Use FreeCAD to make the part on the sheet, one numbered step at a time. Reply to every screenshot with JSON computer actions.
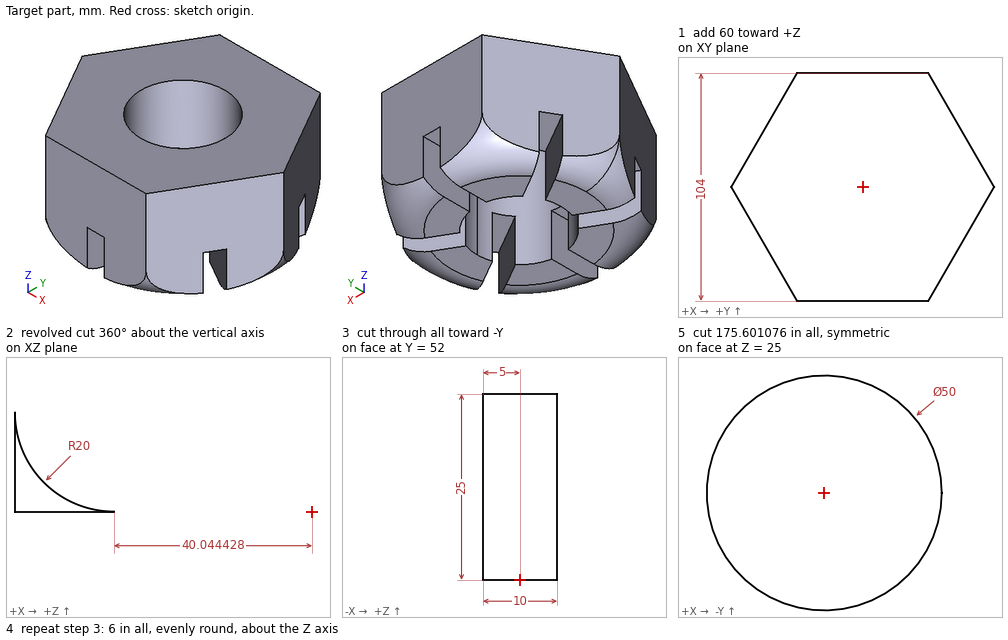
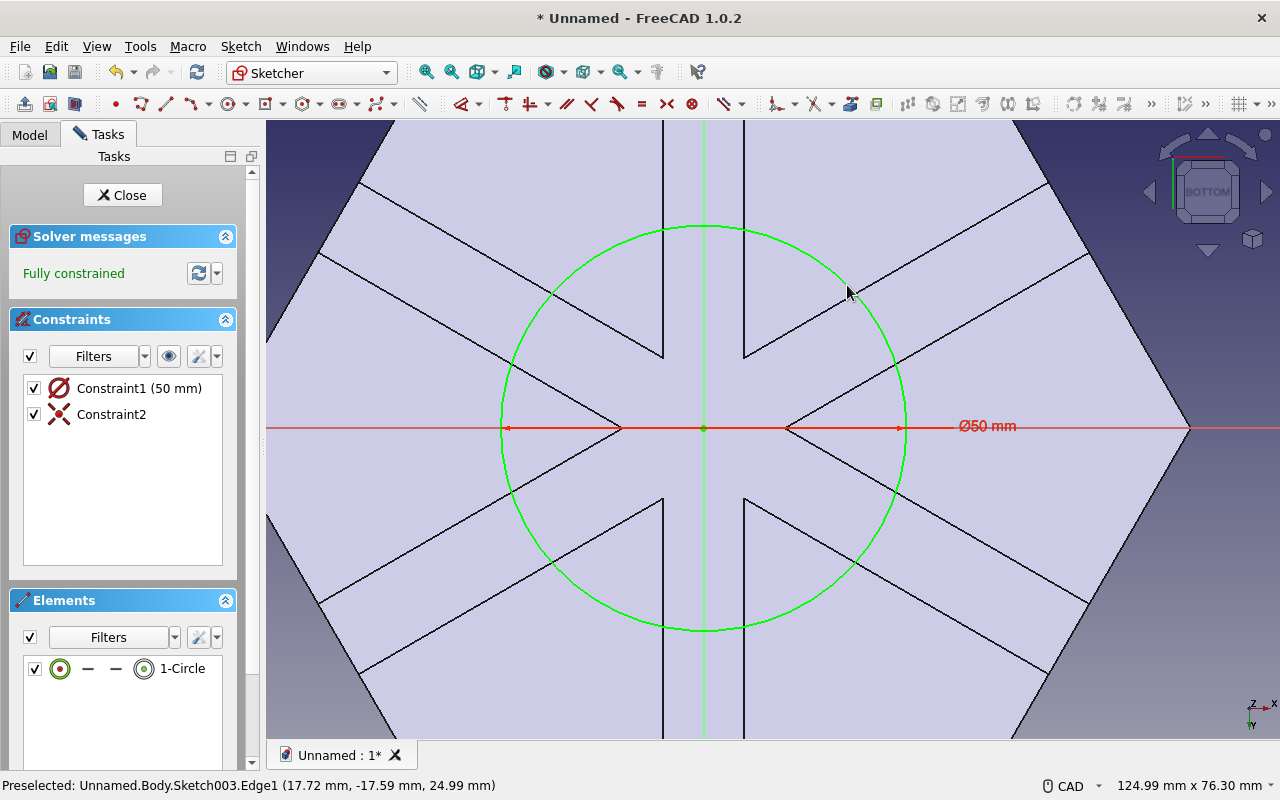
{"action": "left_click", "coordinate": [123, 195]}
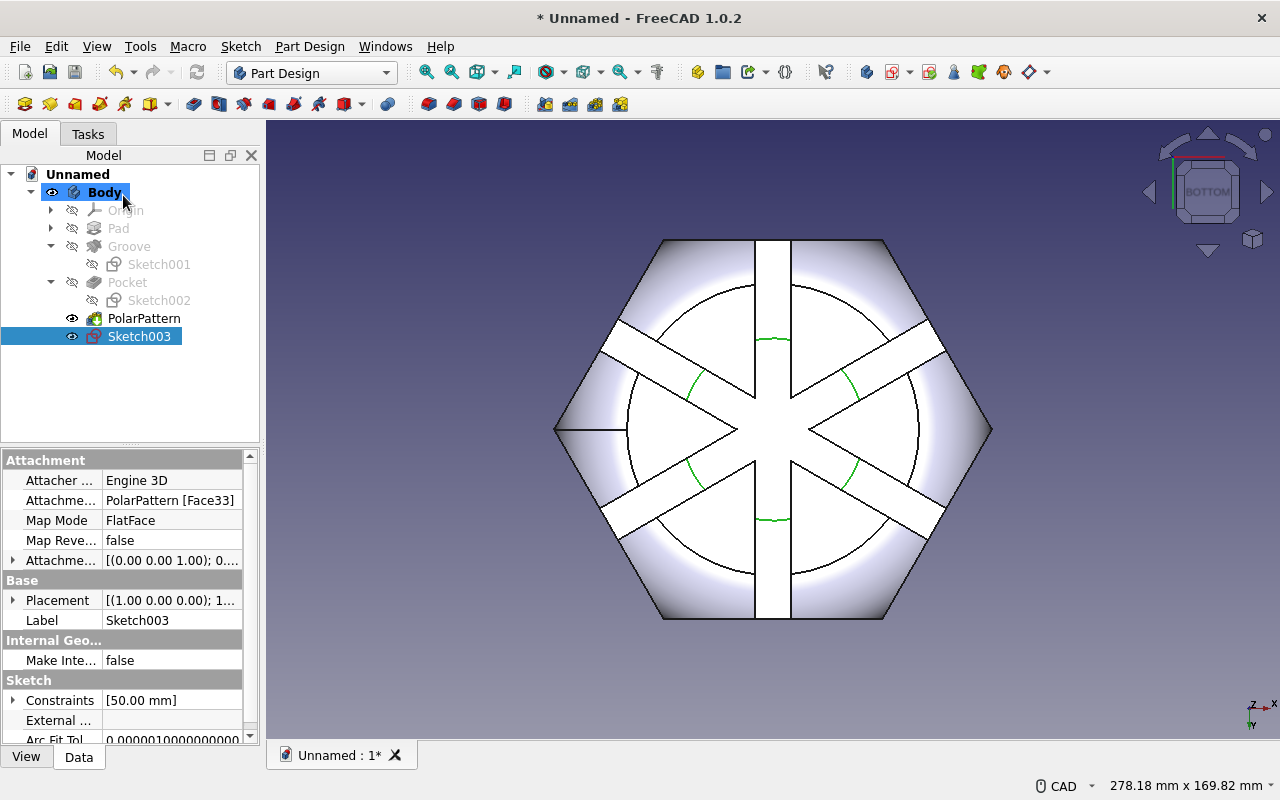
{"action": "left_click", "coordinate": [194, 104]}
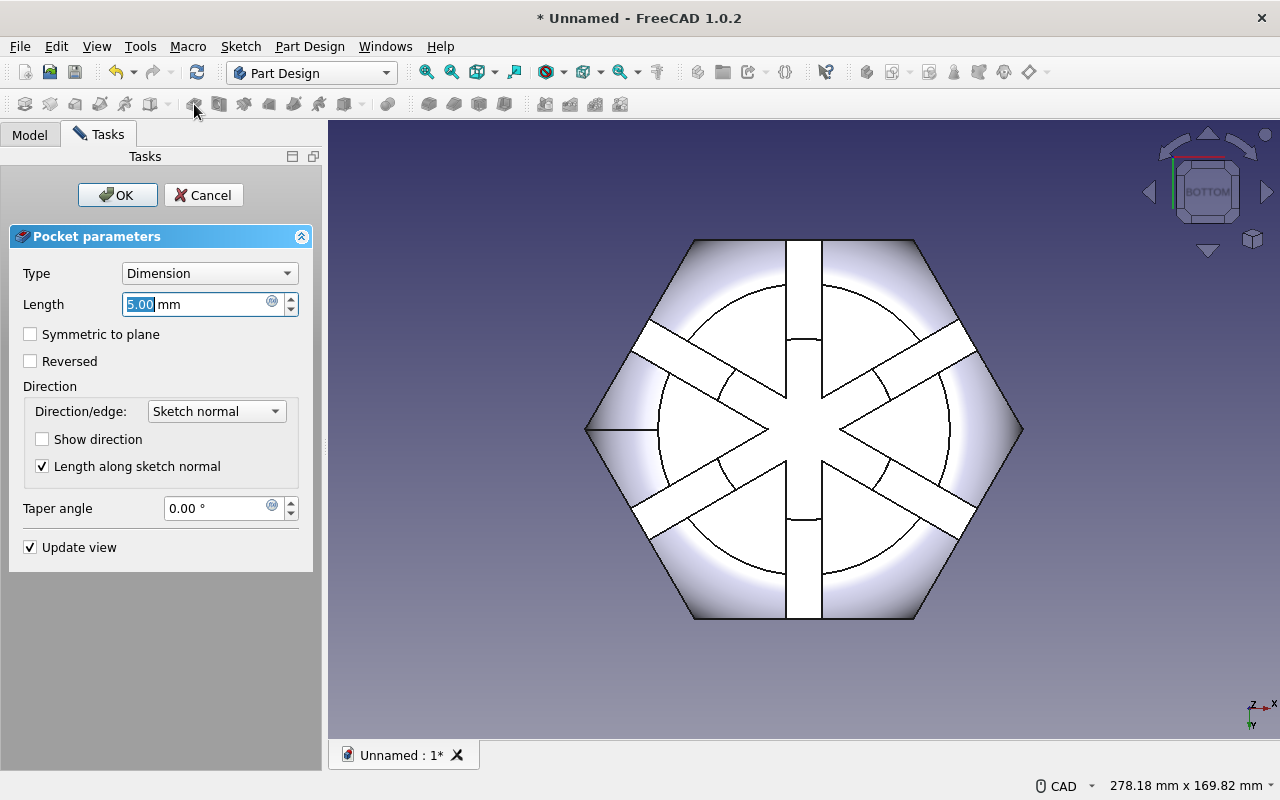
{"action": "type", "text": "175.601076"}
{"action": "key", "text": "Tab"}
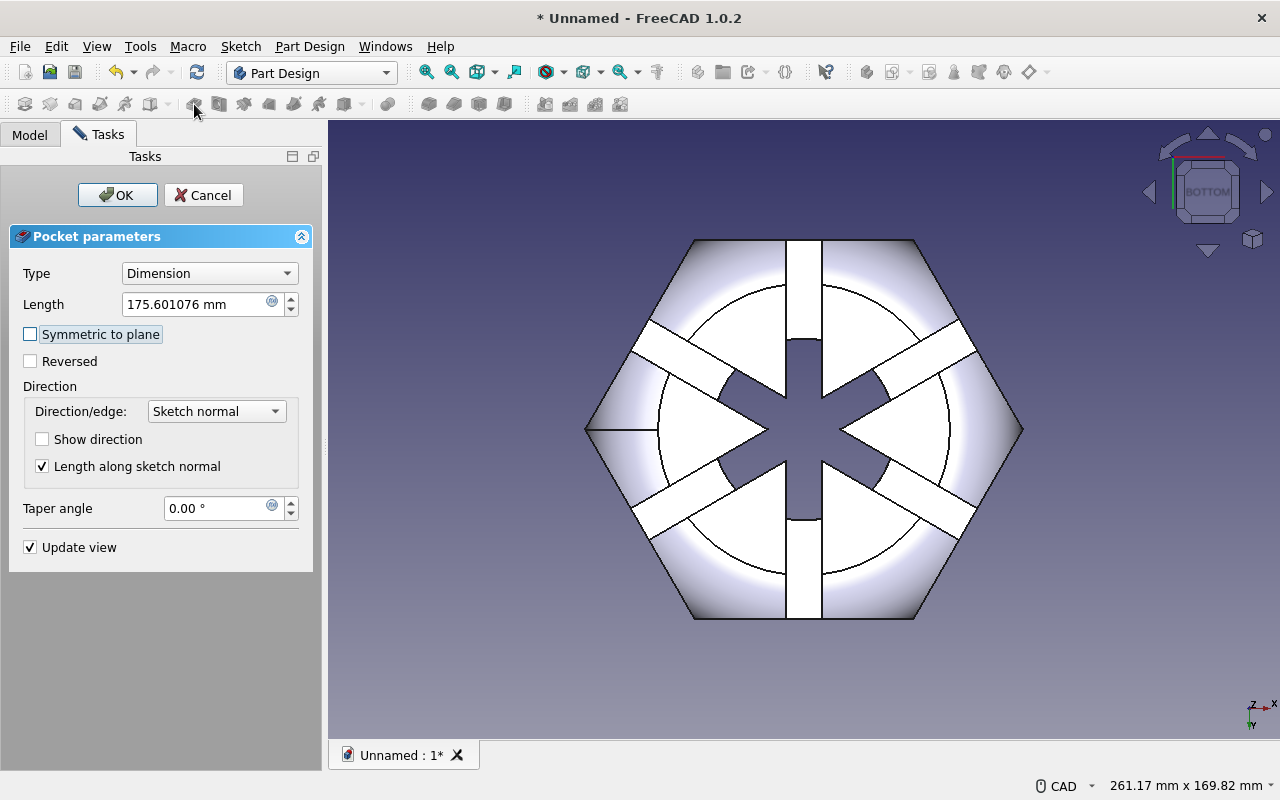
{"action": "left_click", "coordinate": [31, 334]}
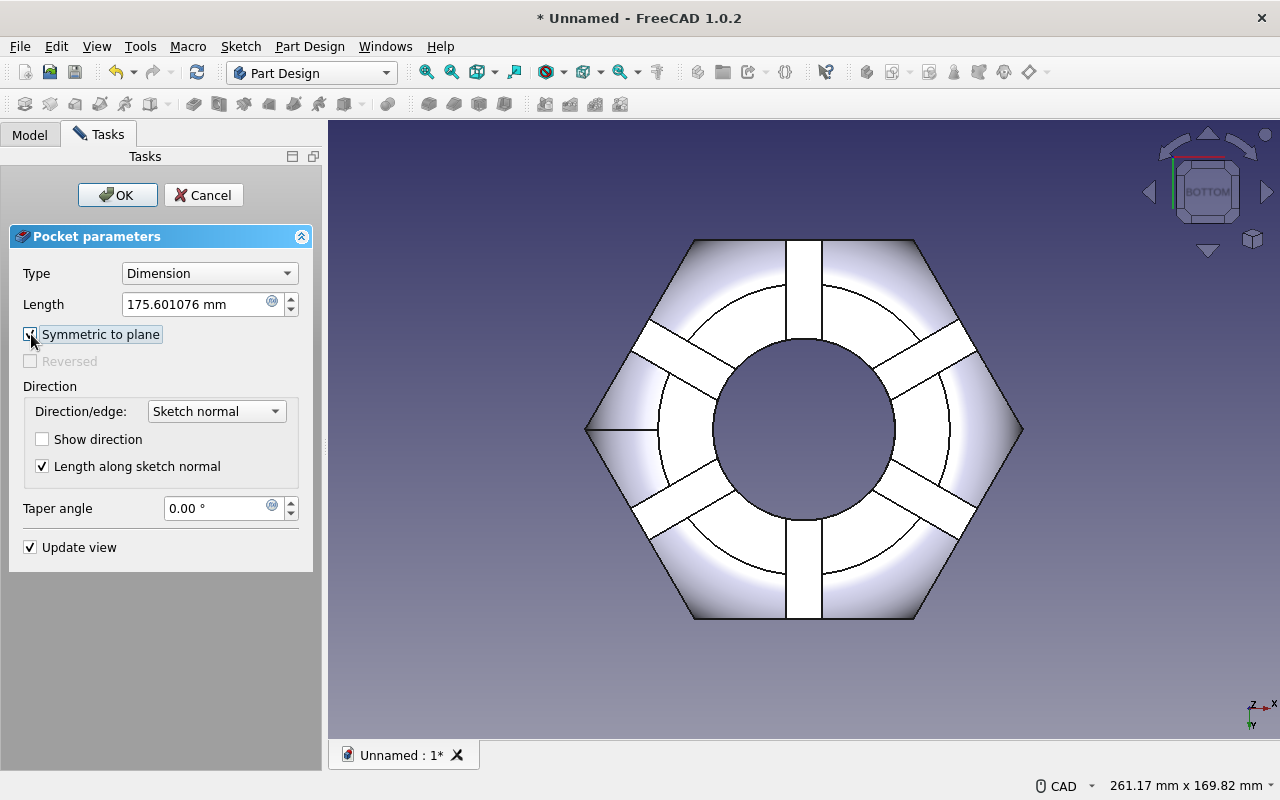
{"action": "left_click", "coordinate": [118, 195]}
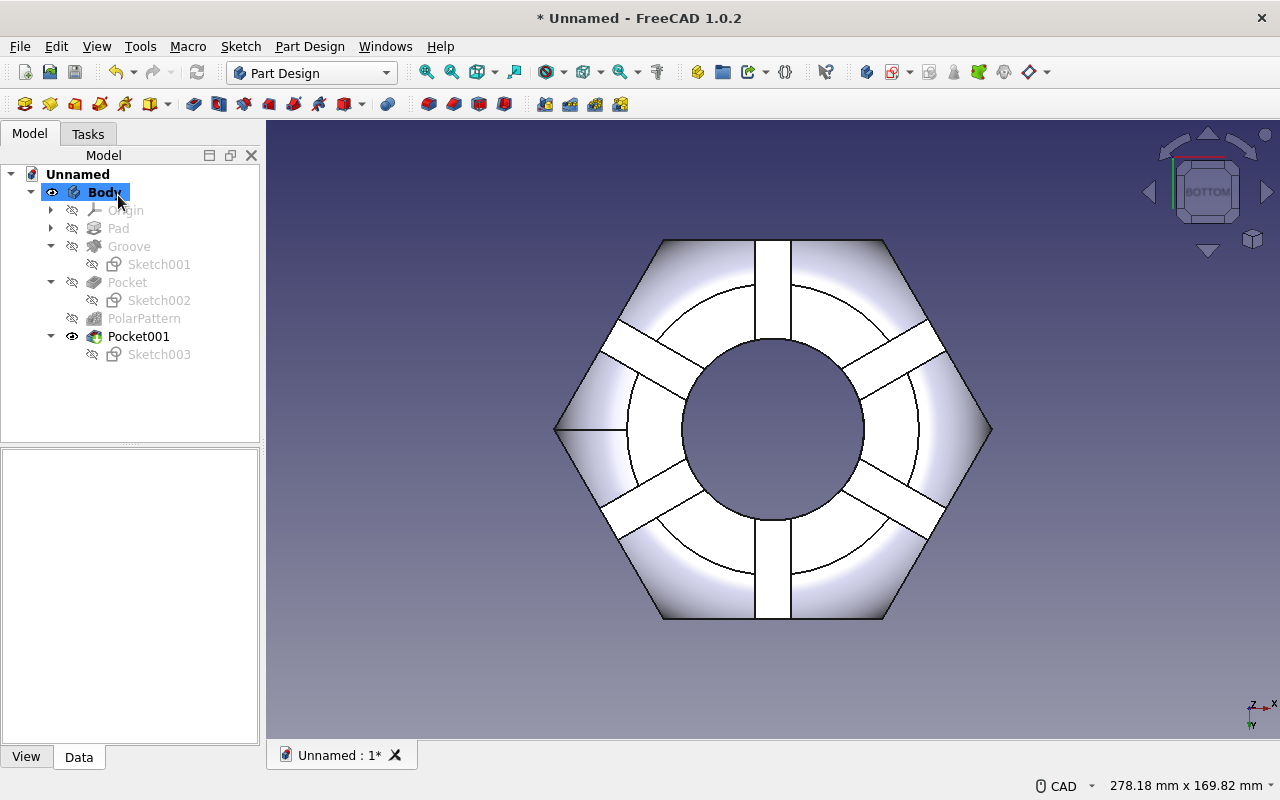
{"action": "key", "text": "0"}